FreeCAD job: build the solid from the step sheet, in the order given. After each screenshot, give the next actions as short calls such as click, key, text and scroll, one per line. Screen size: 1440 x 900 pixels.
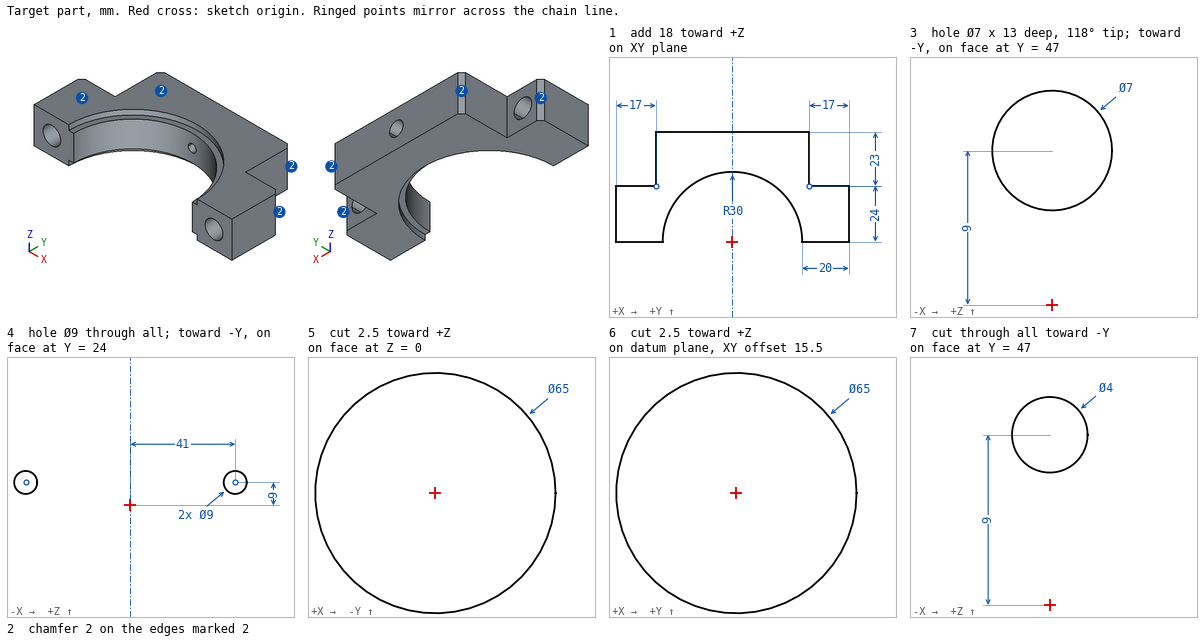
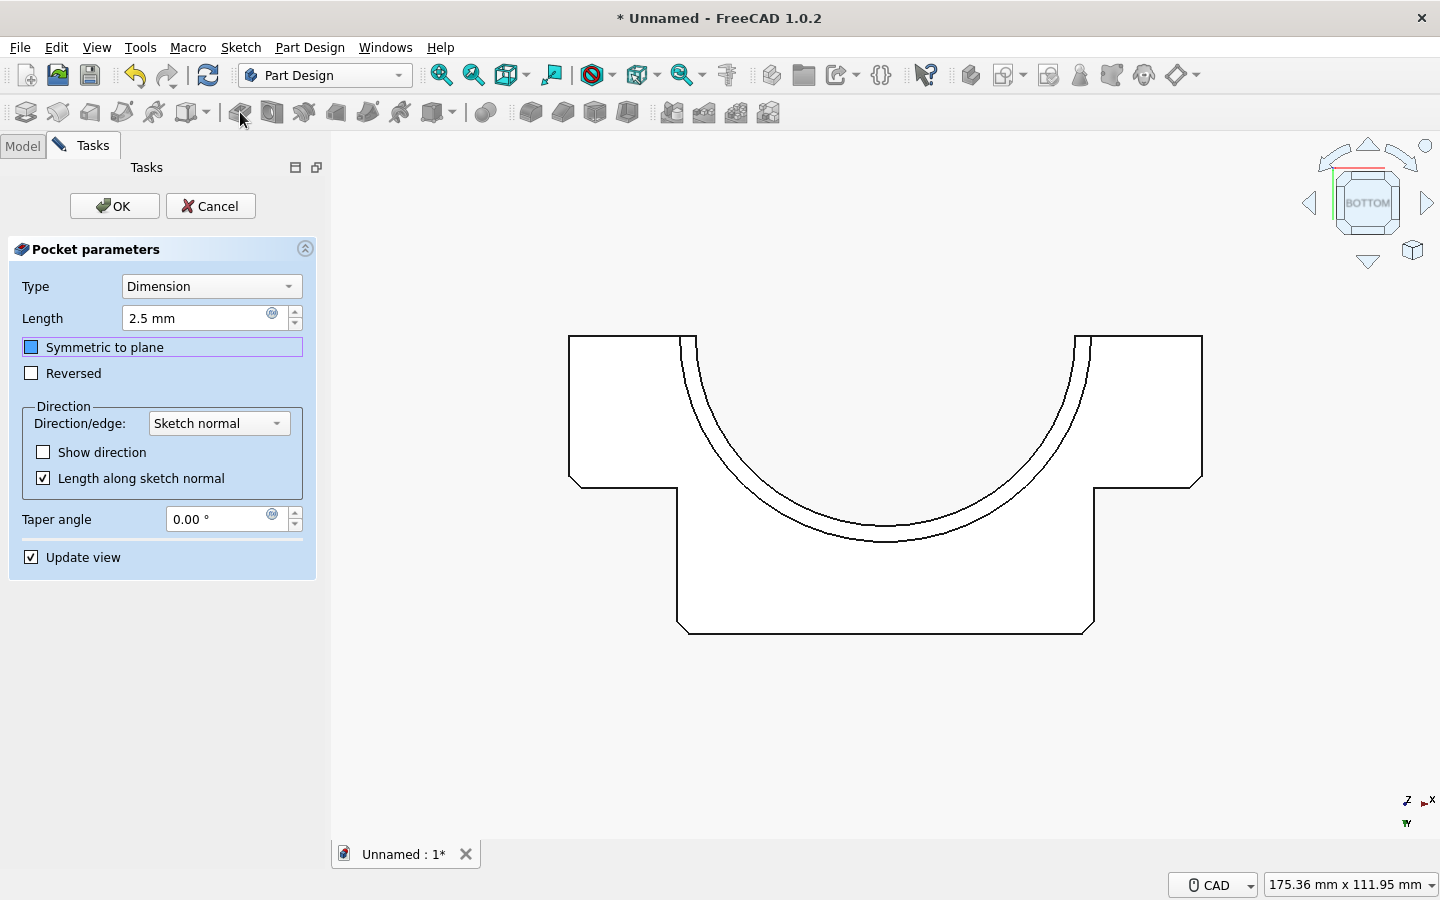
click(115, 206)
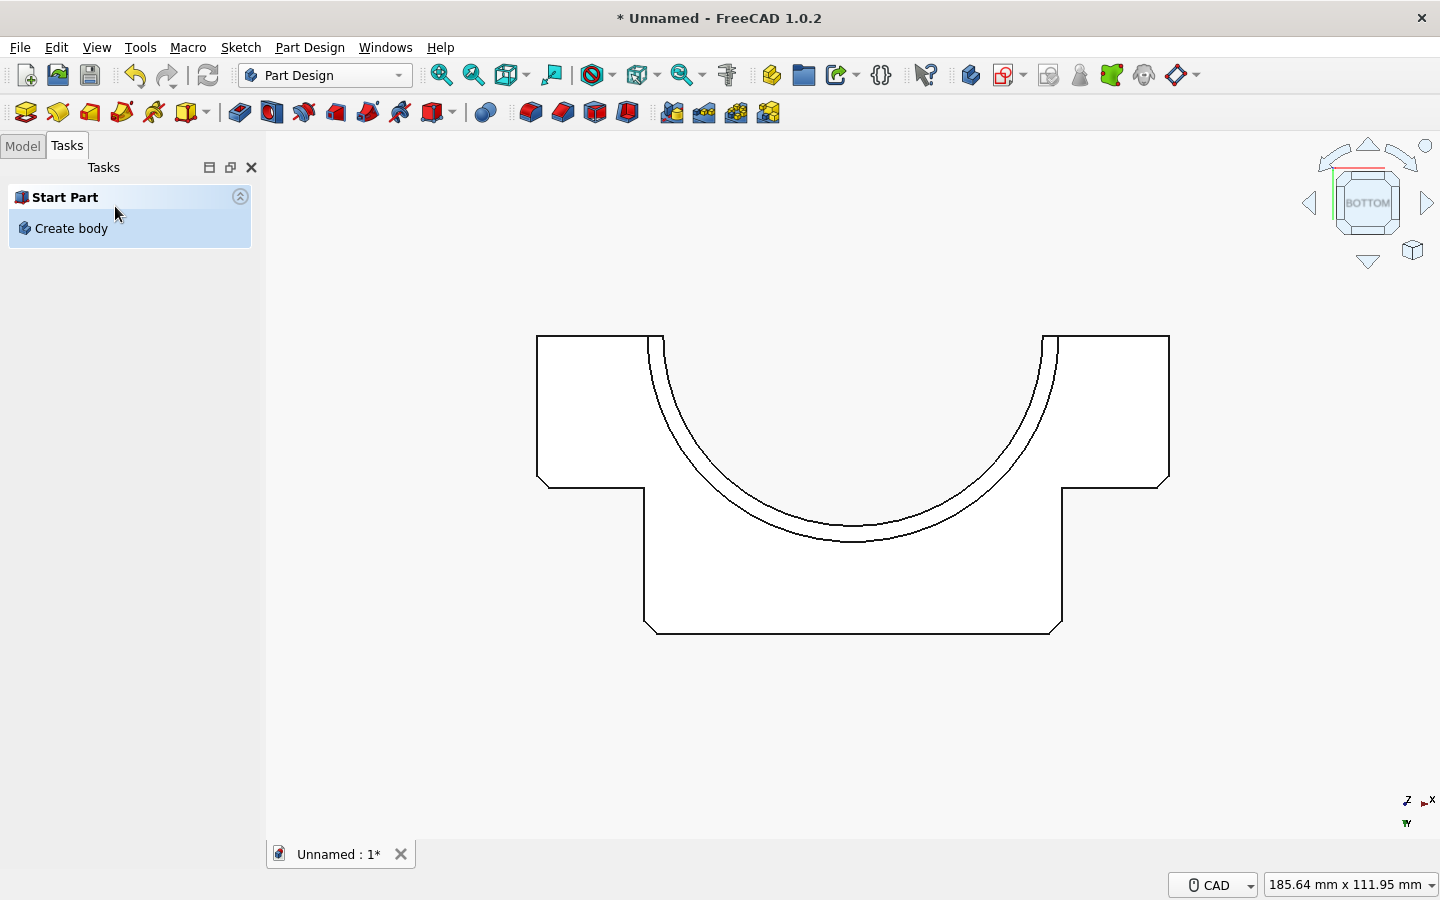
click(23, 145)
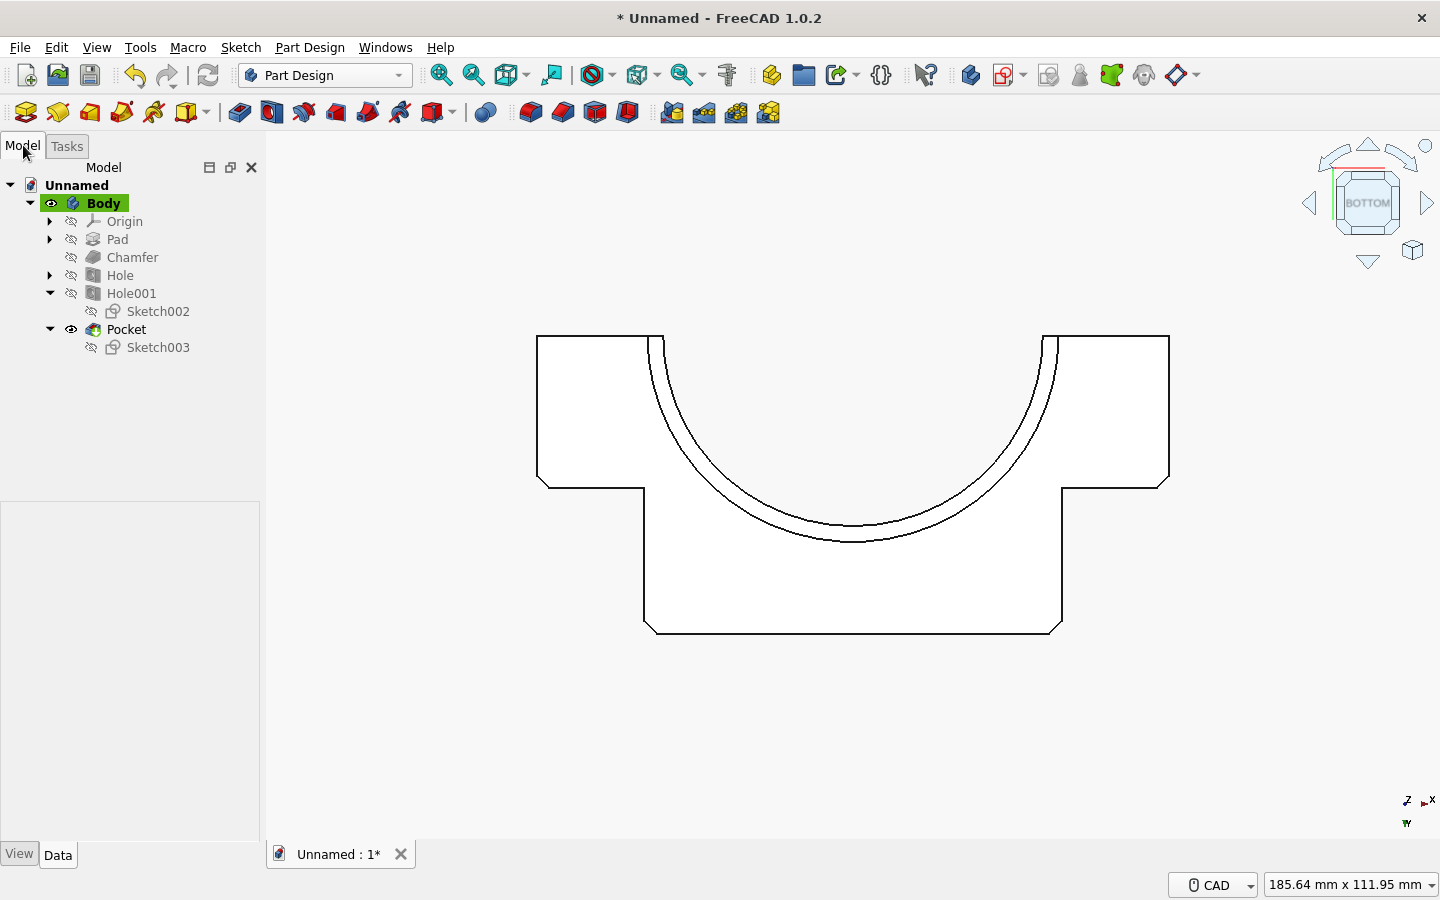
click(50, 221)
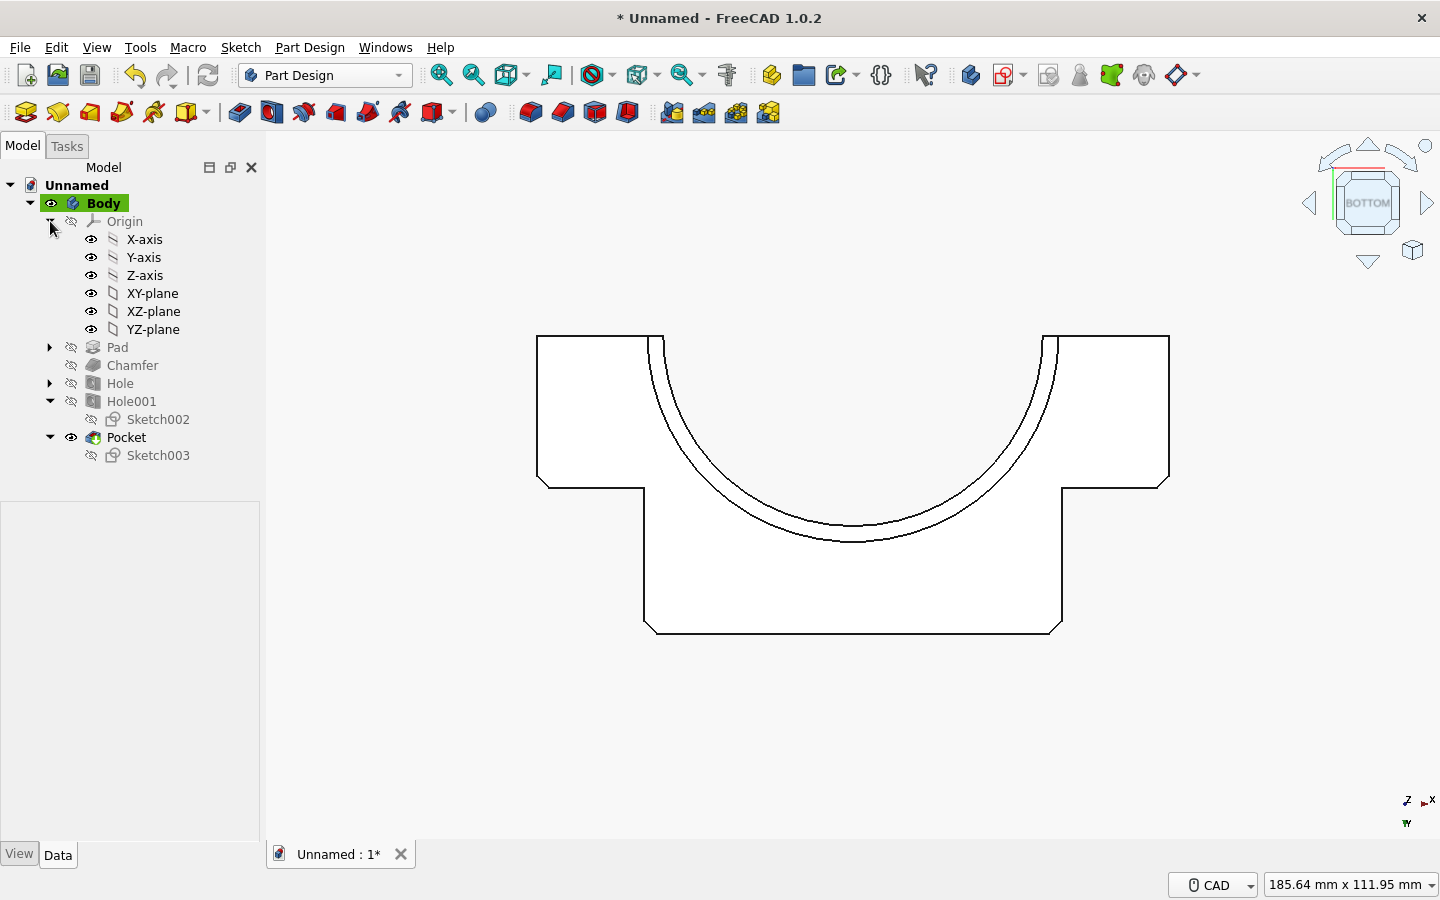
click(136, 293)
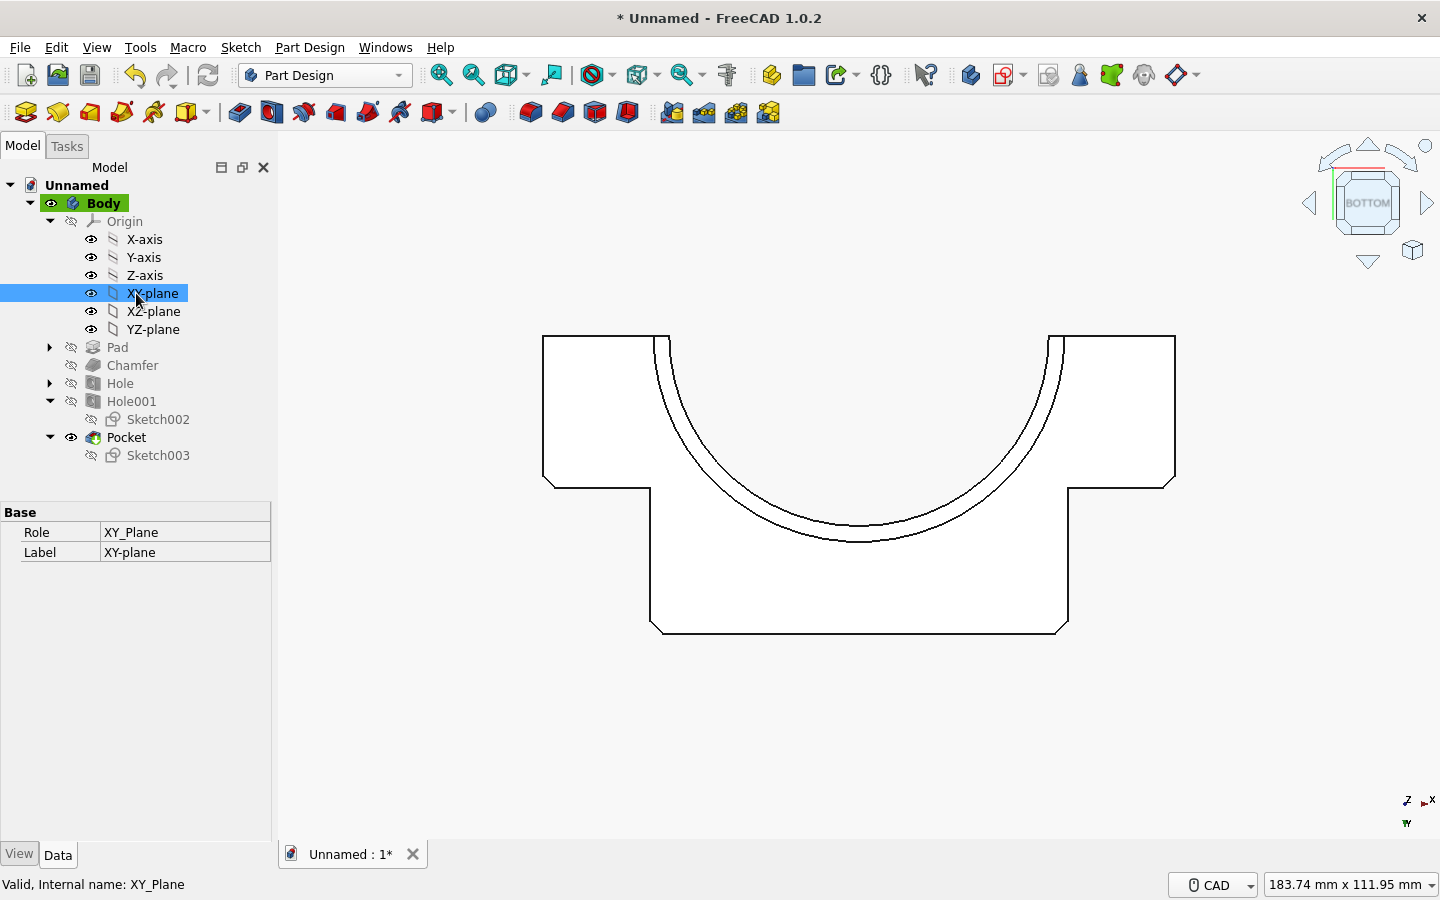
click(1176, 76)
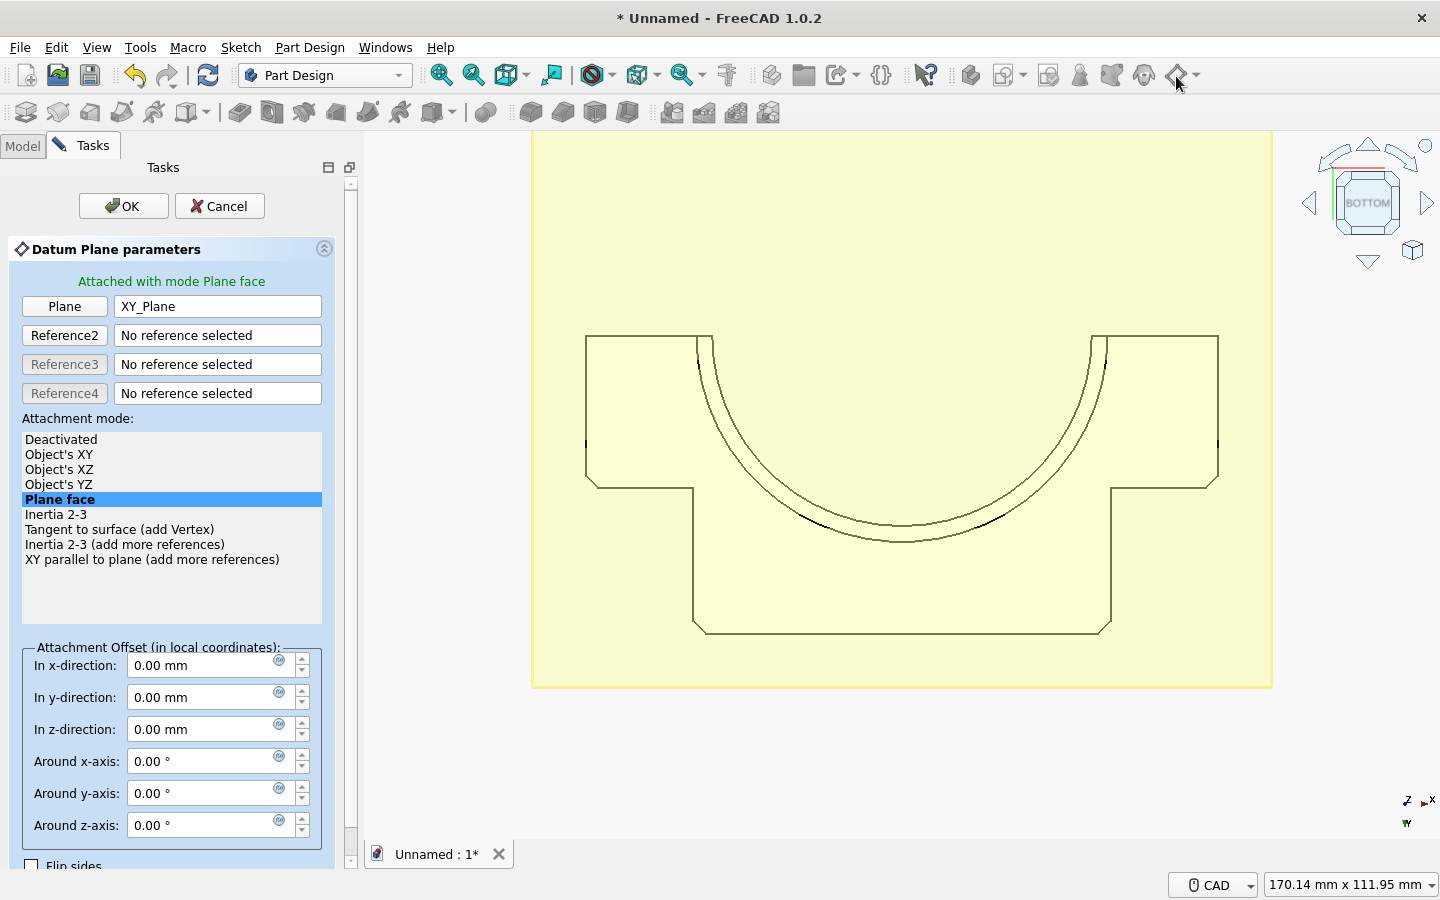
triple_click(210, 729)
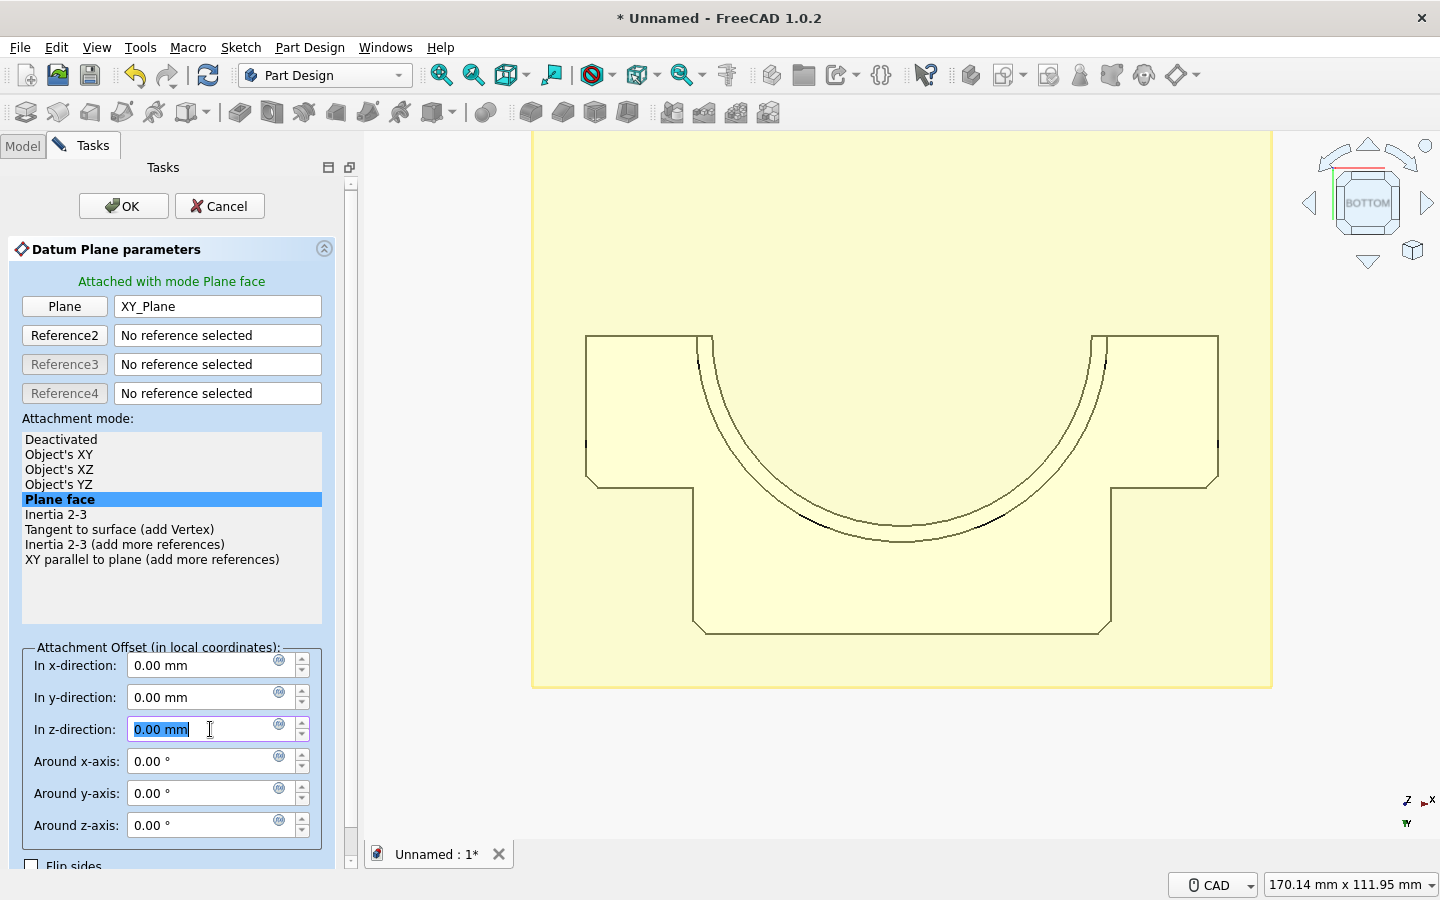
text(15.5)
key(Tab)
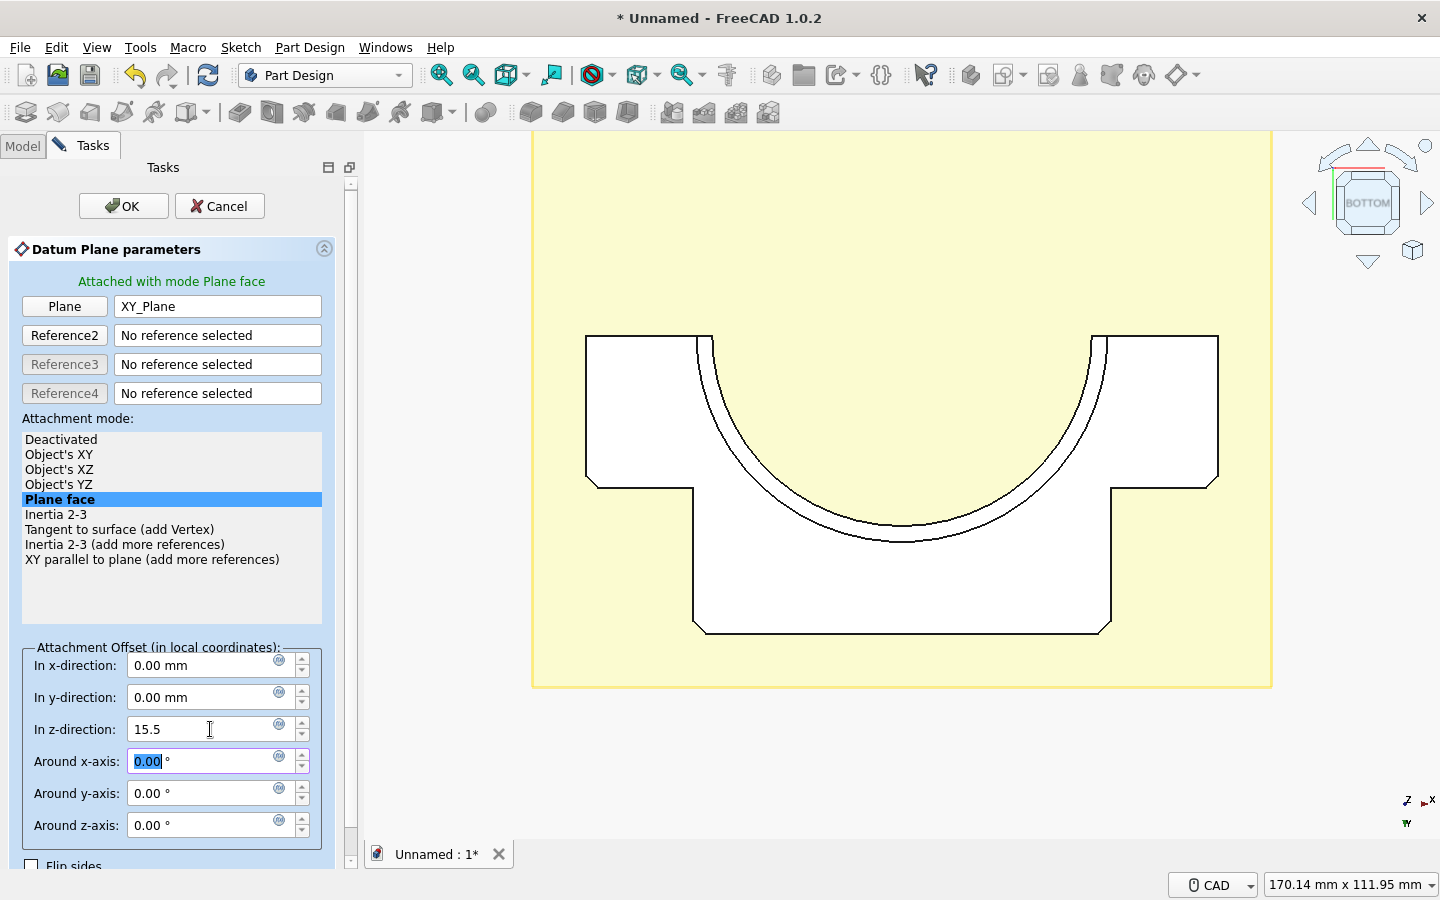
click(124, 206)